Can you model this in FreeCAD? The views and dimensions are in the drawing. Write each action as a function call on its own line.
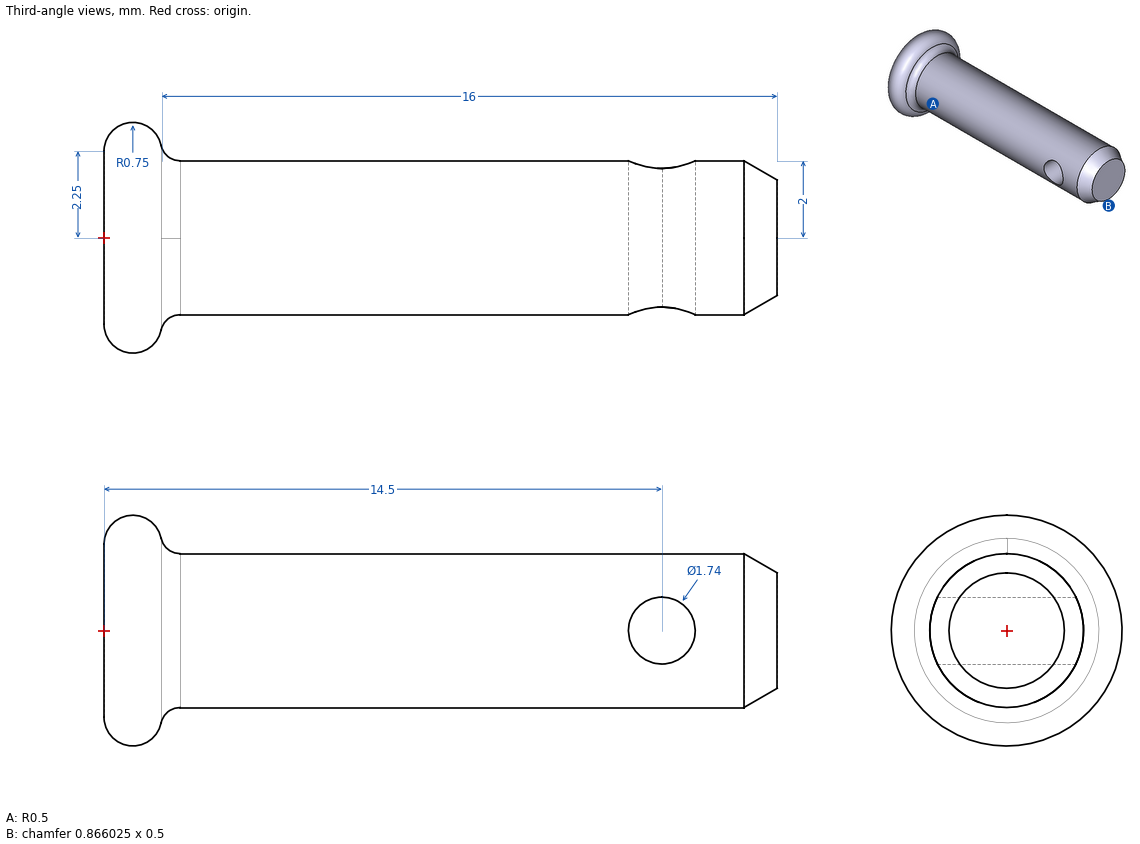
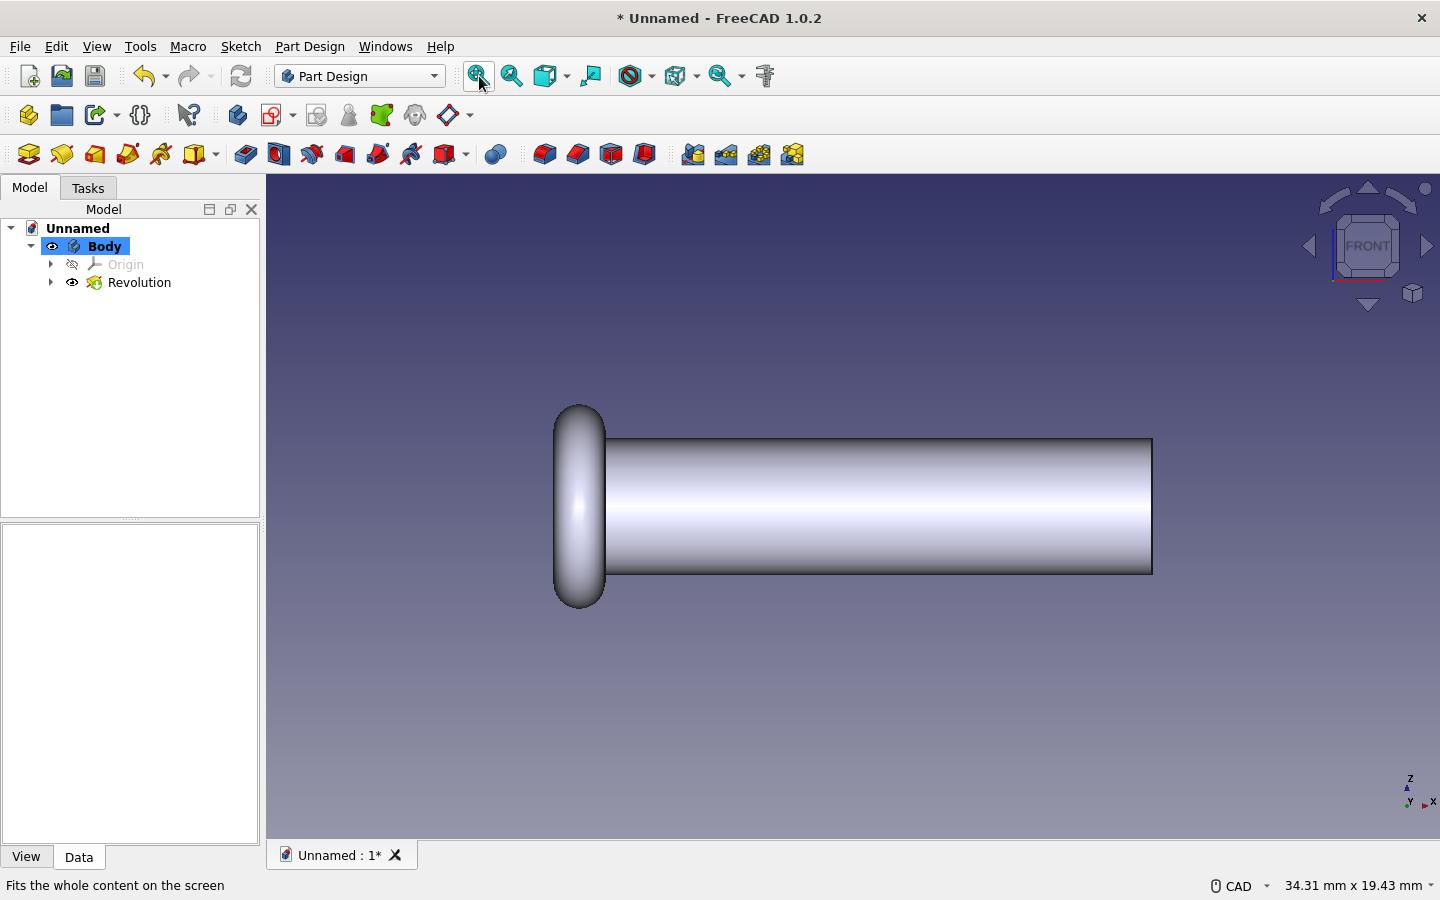
key(3)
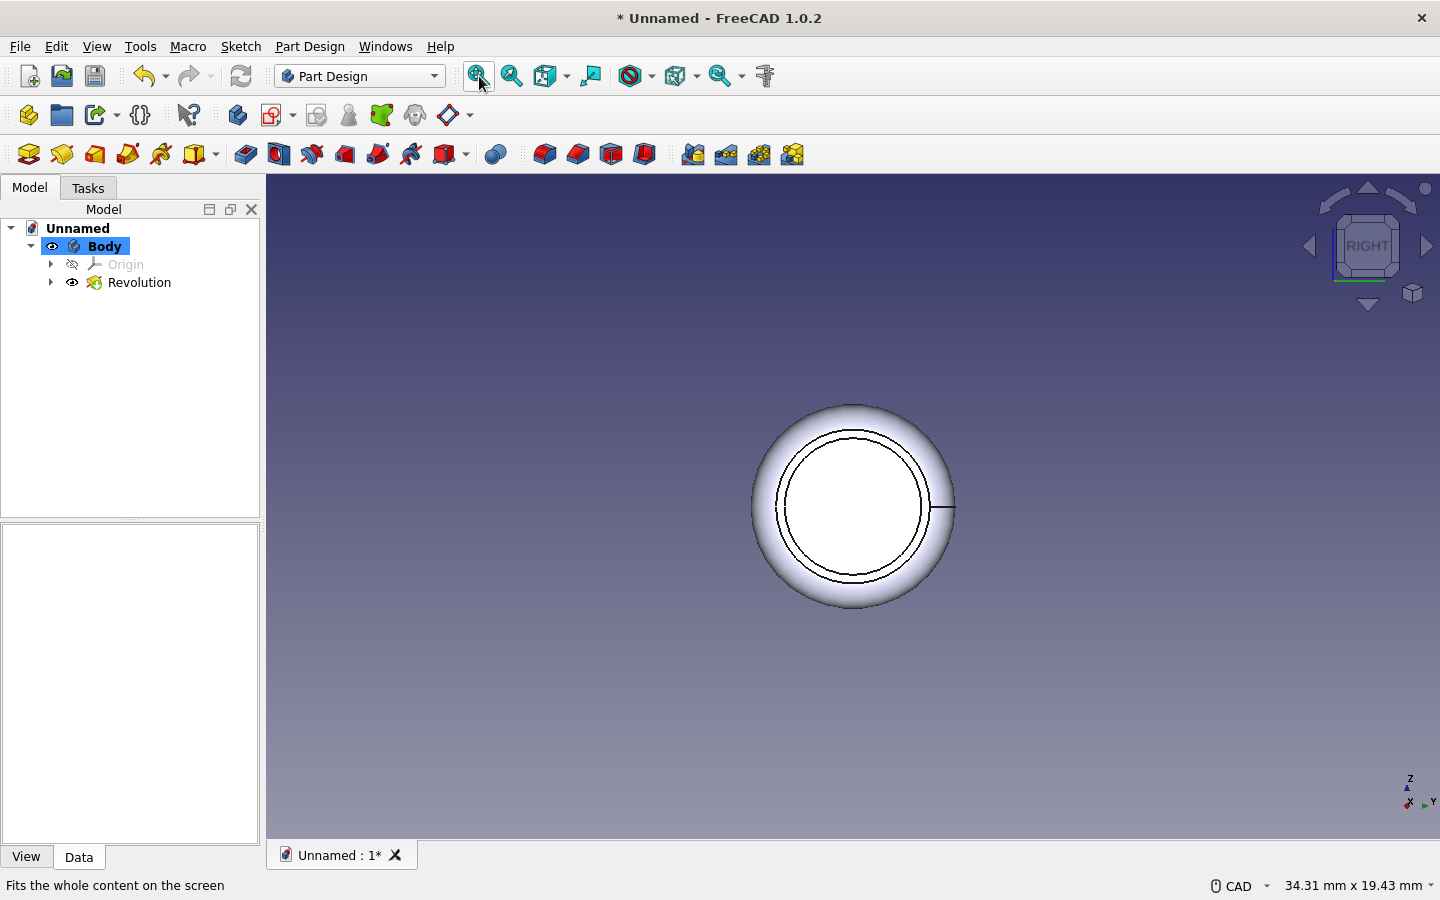
click(479, 76)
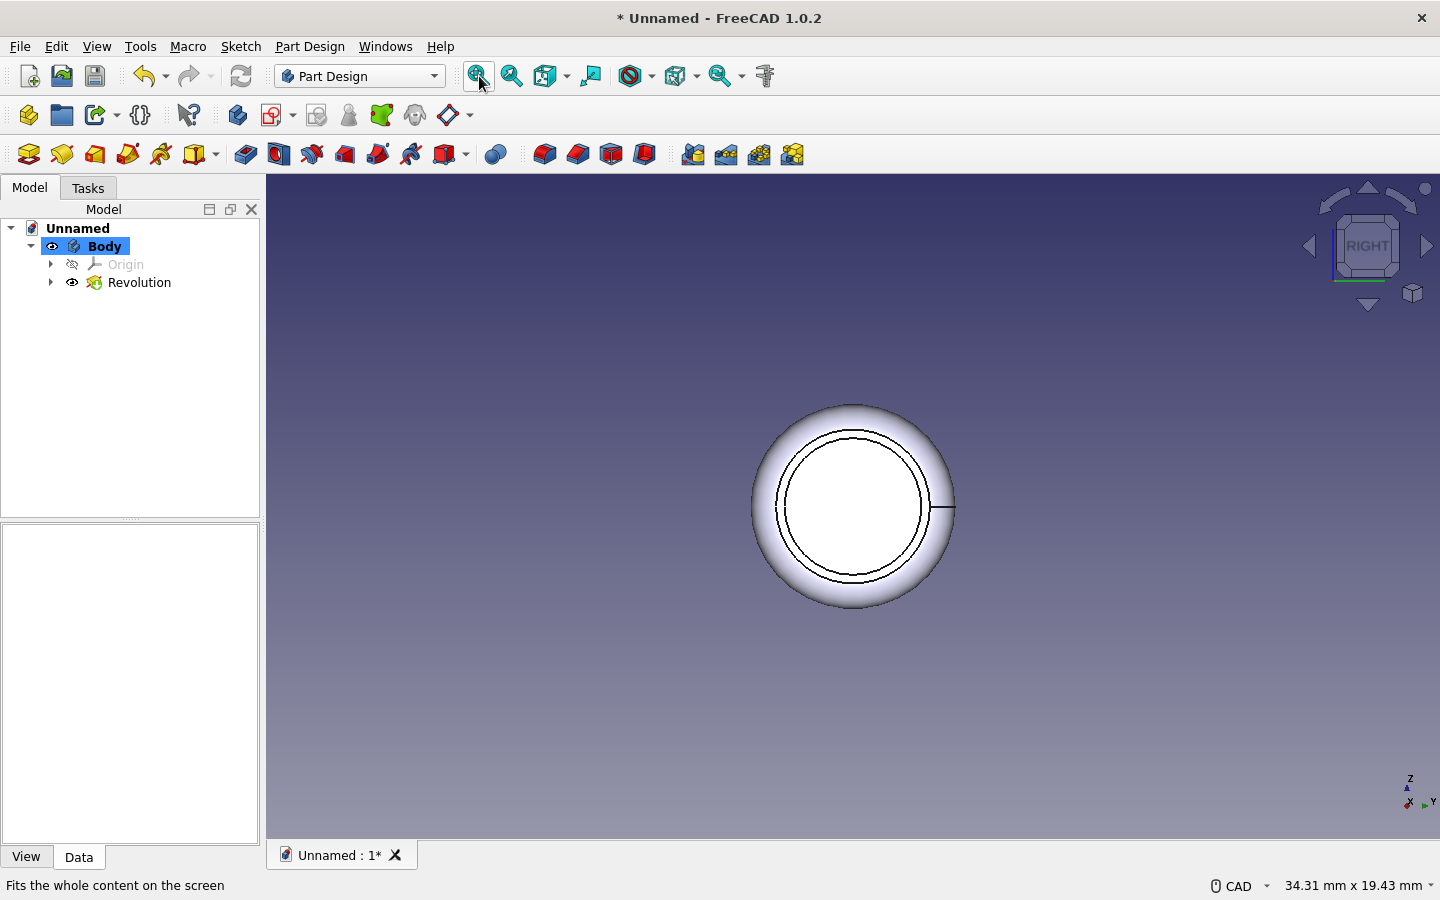
key(5)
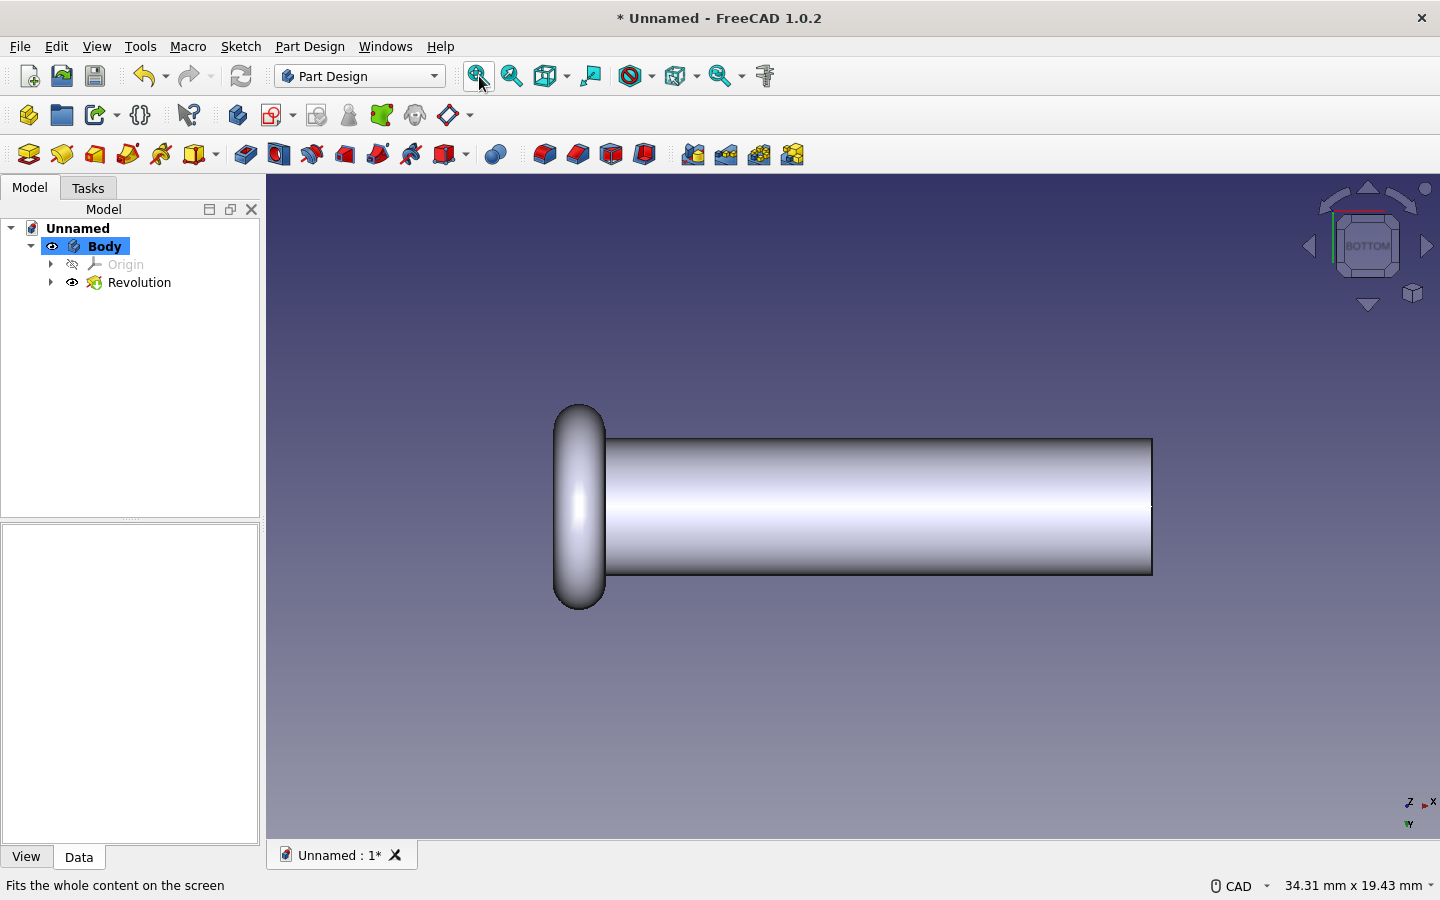
key(4)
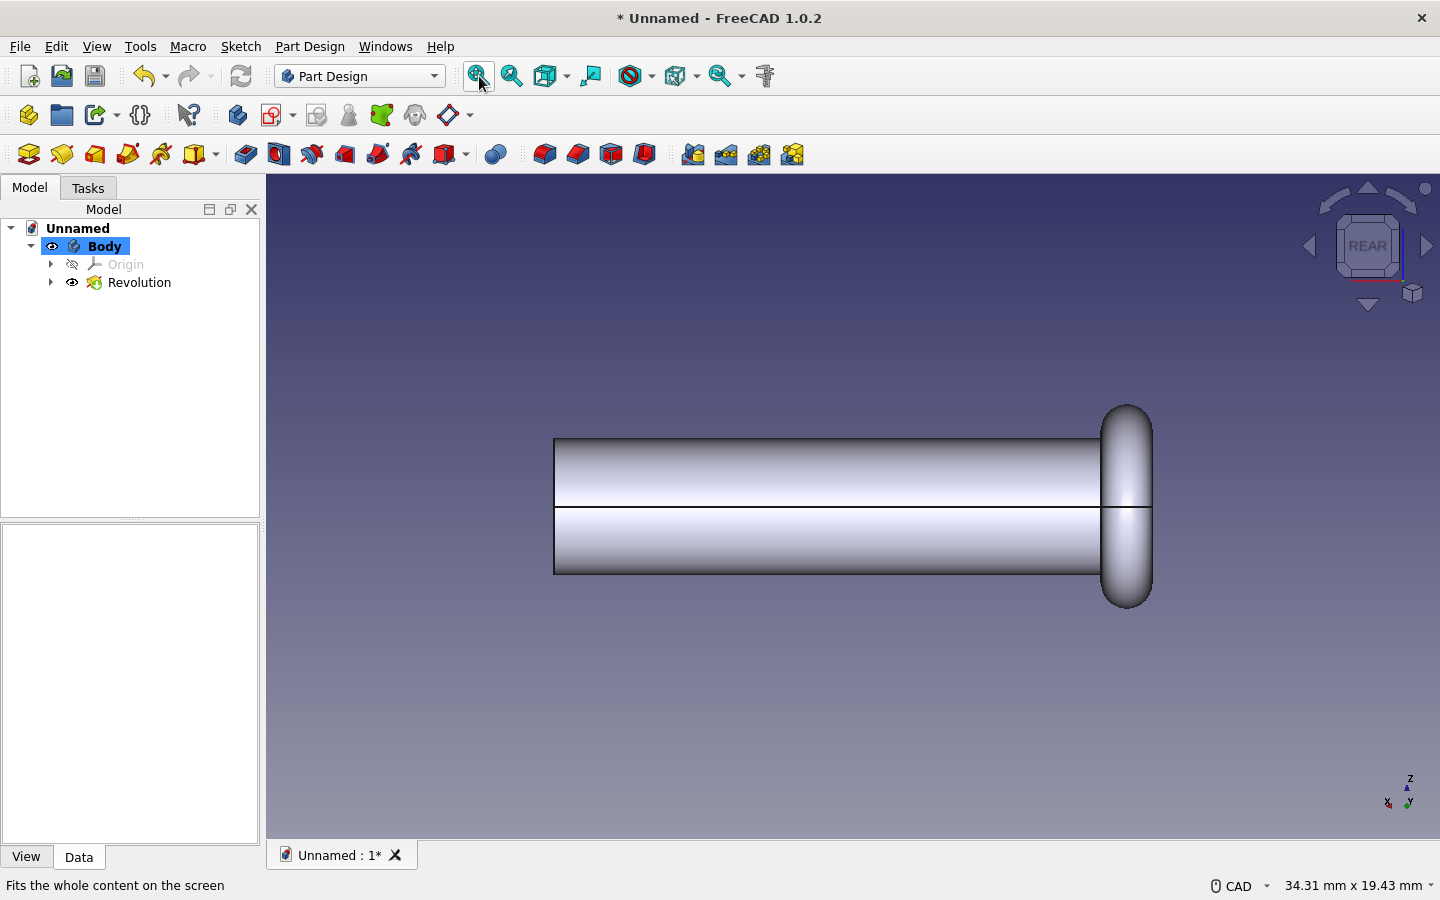
key(6)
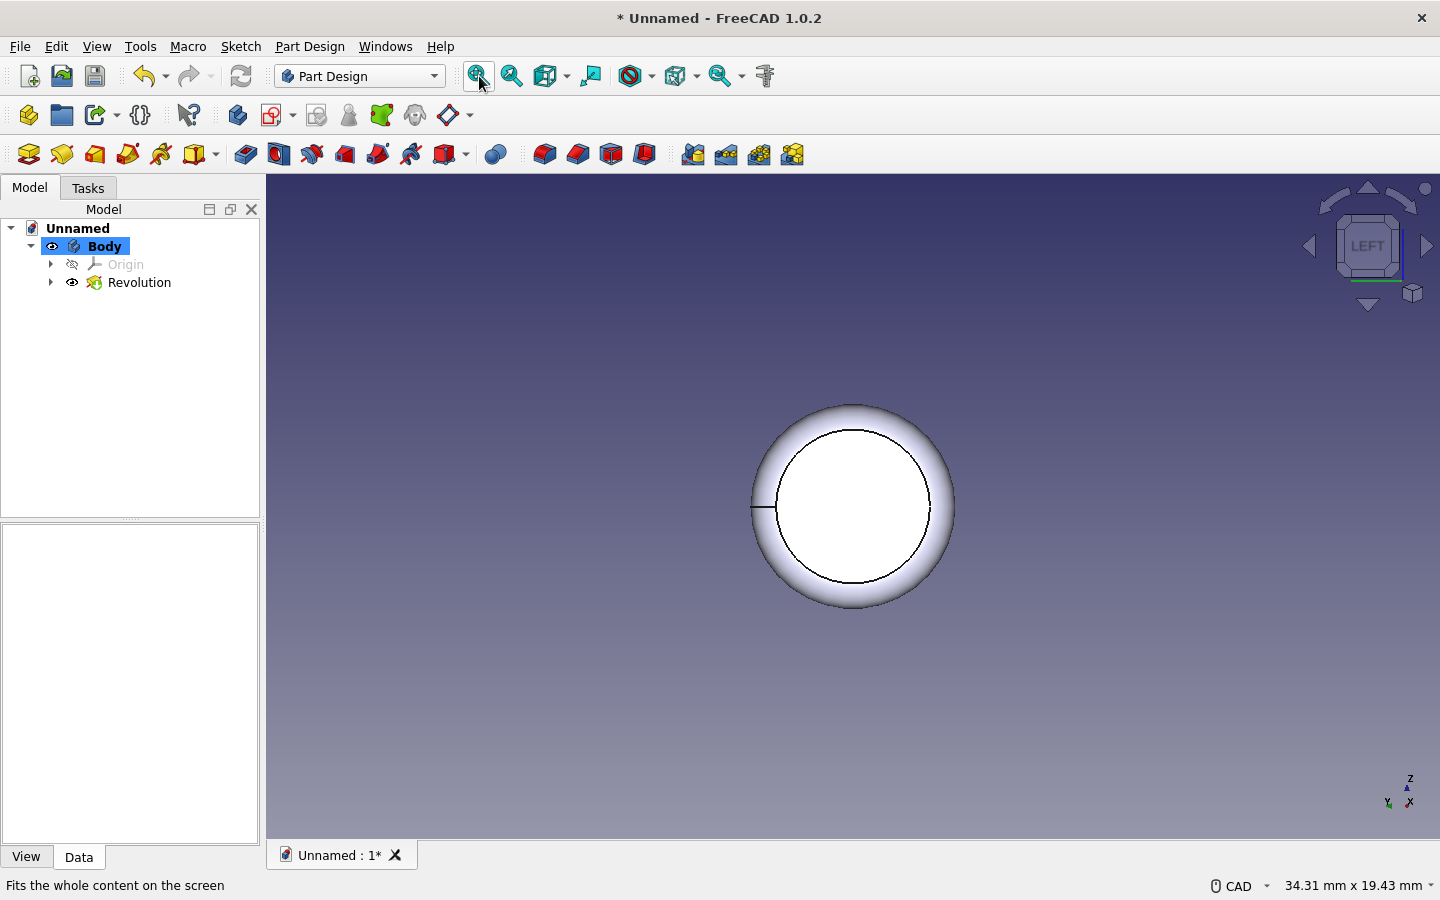
click(479, 76)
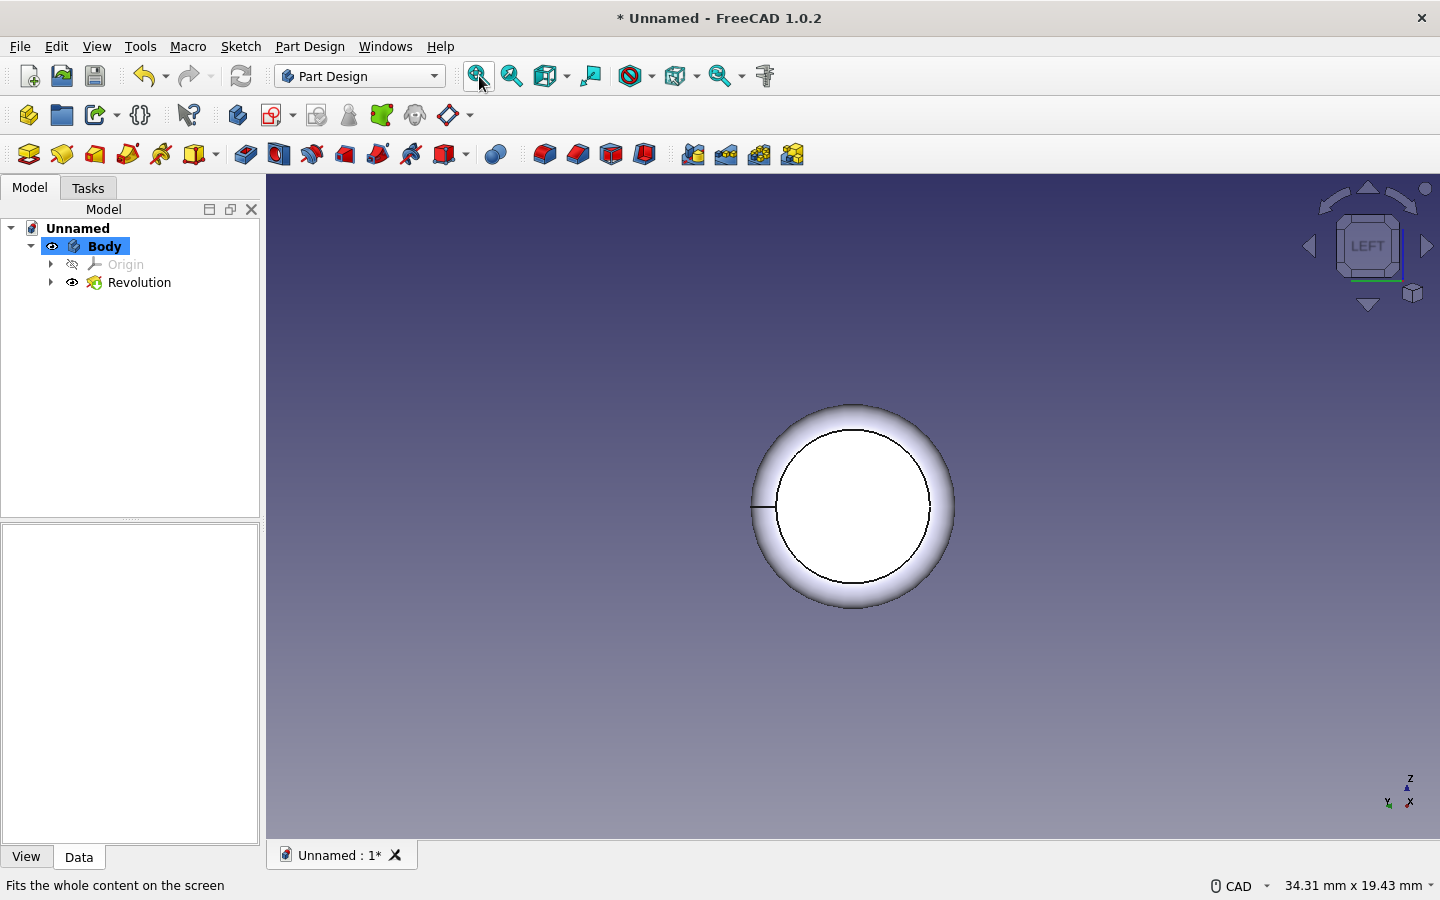
key(v)
key(3)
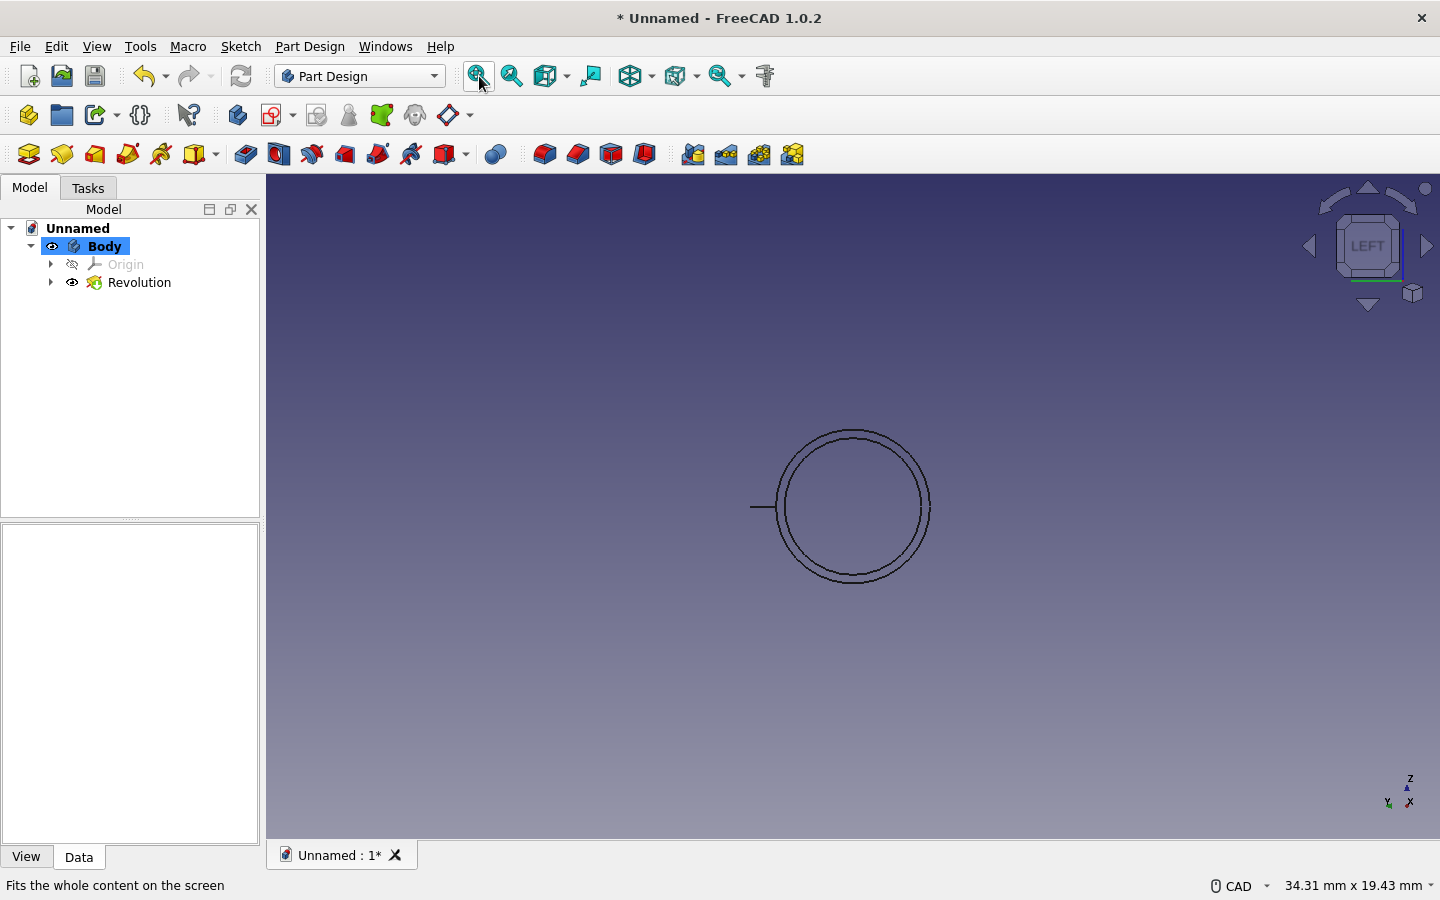
key(0)